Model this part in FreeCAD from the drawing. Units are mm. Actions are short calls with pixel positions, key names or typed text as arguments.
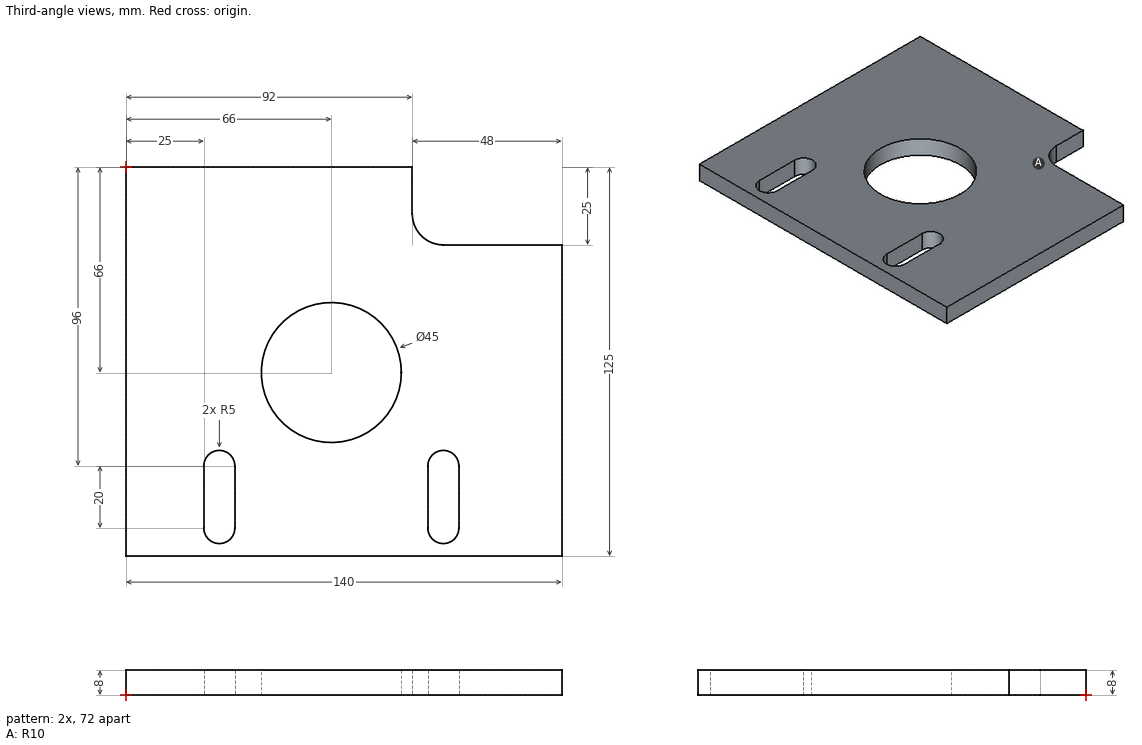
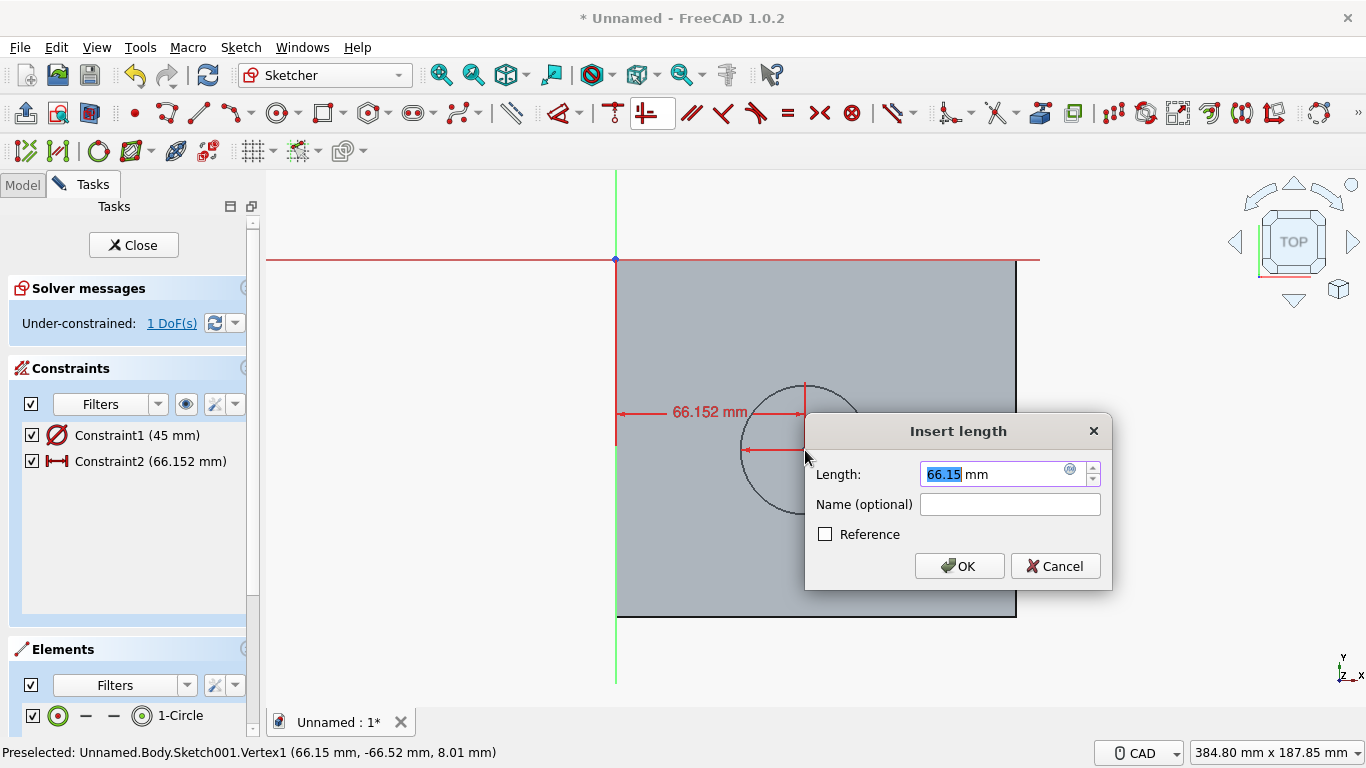
text(66)
key(Return)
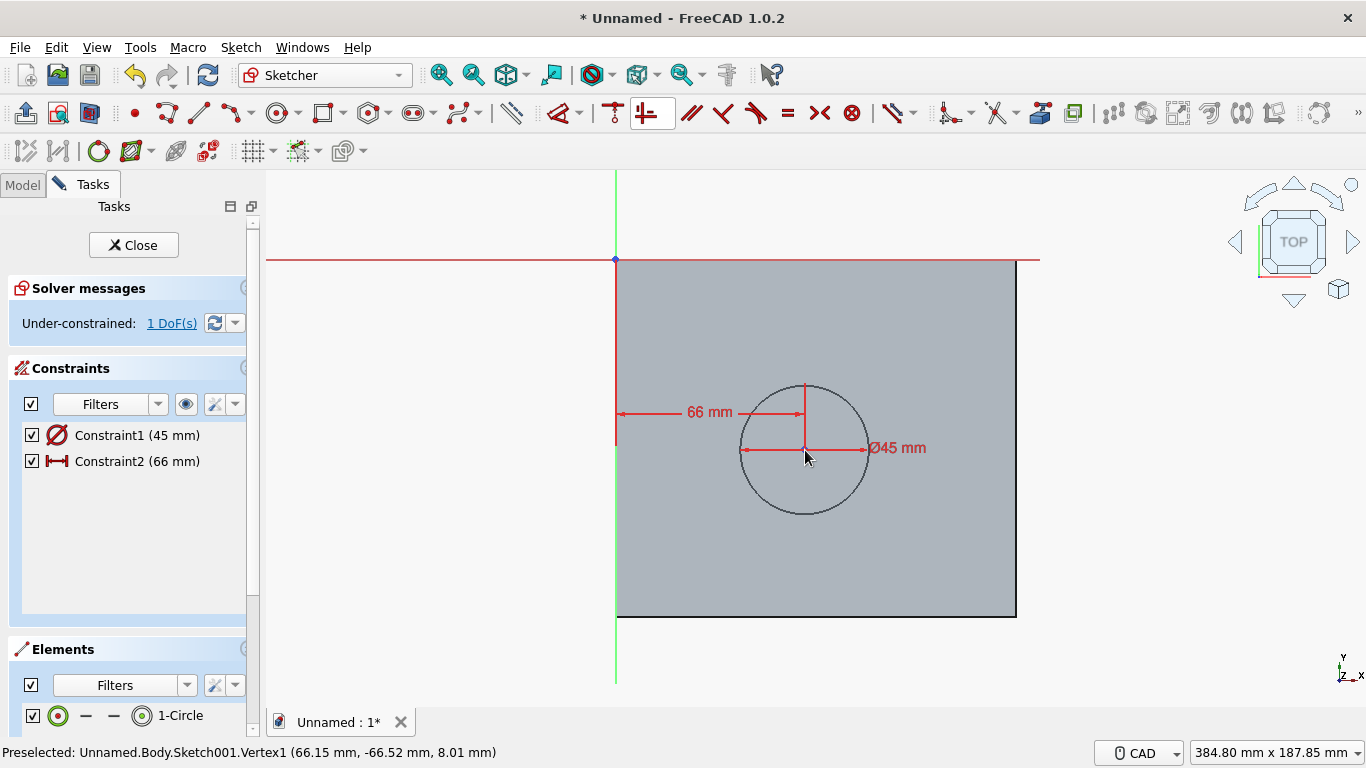
click(805, 450)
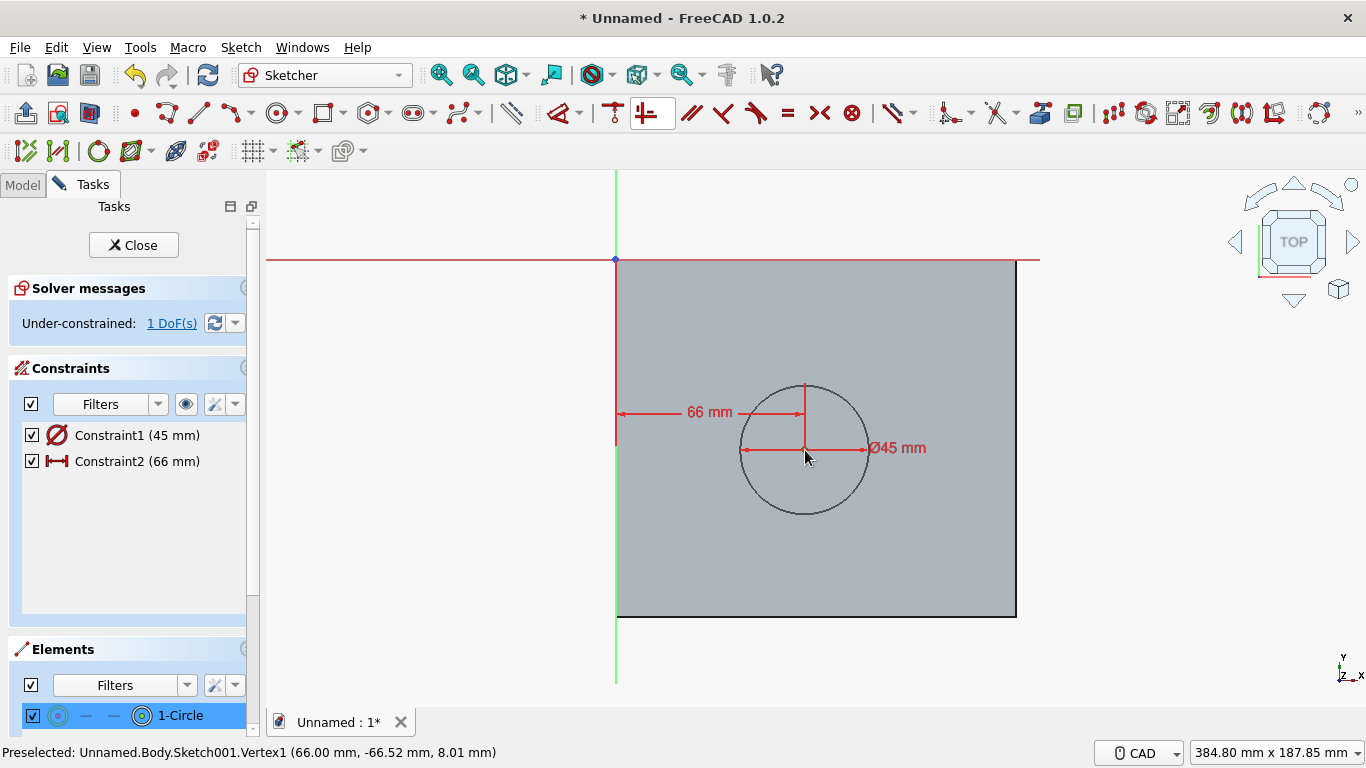
key(i)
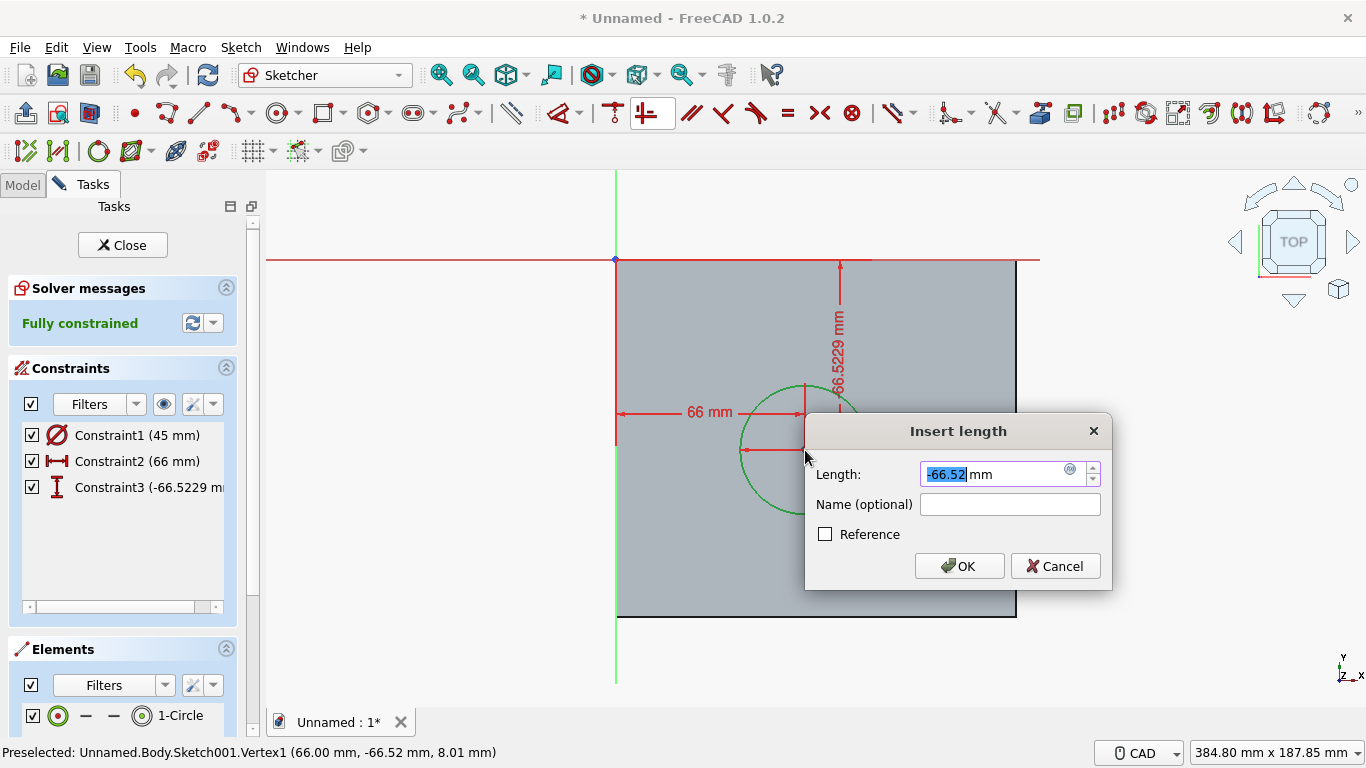
text(-66)
key(Return)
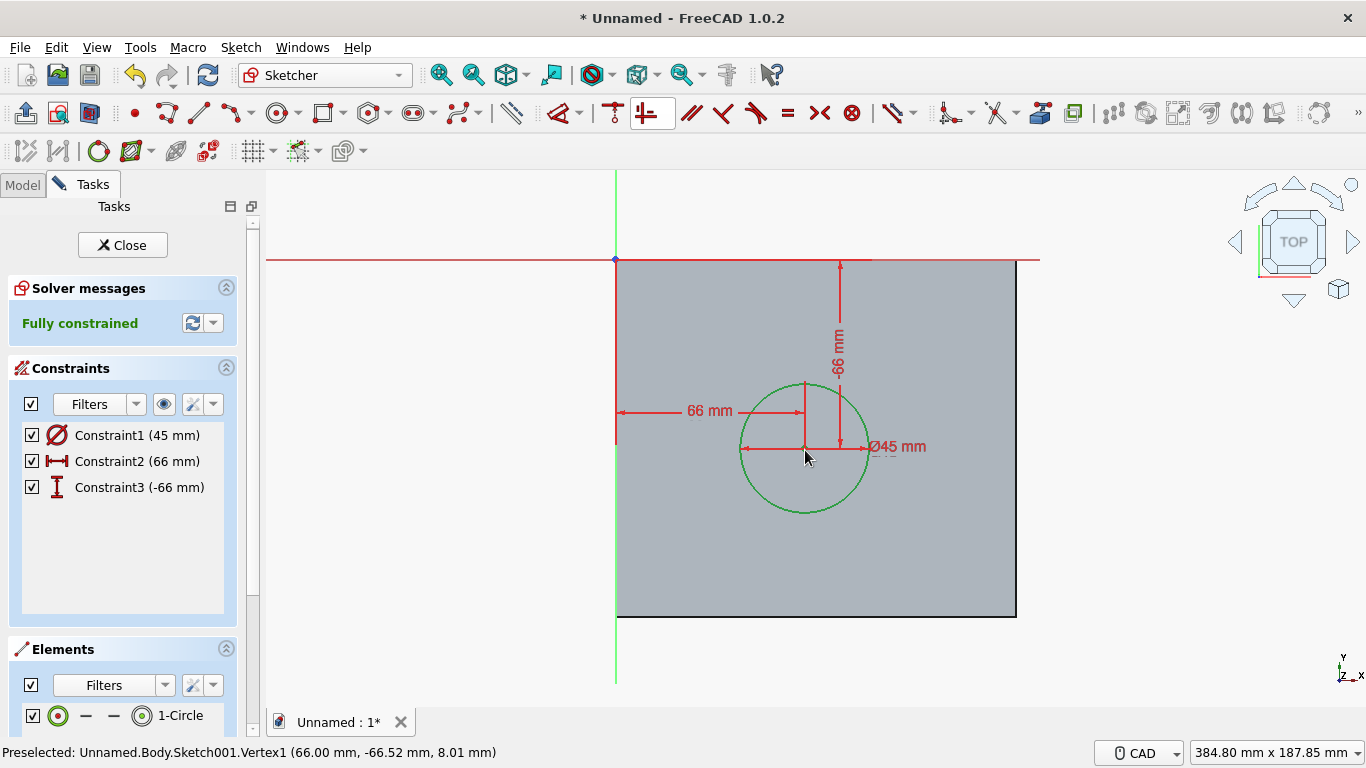
click(123, 245)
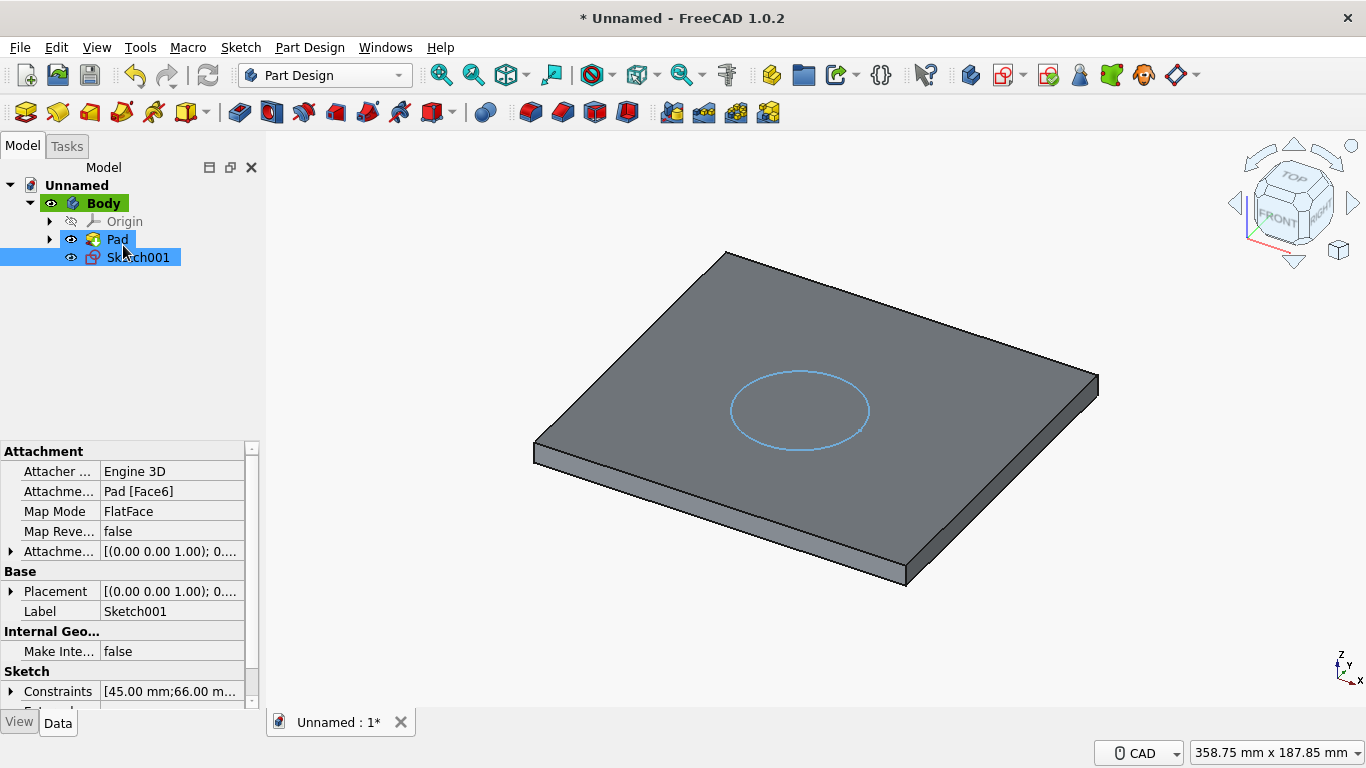
click(240, 112)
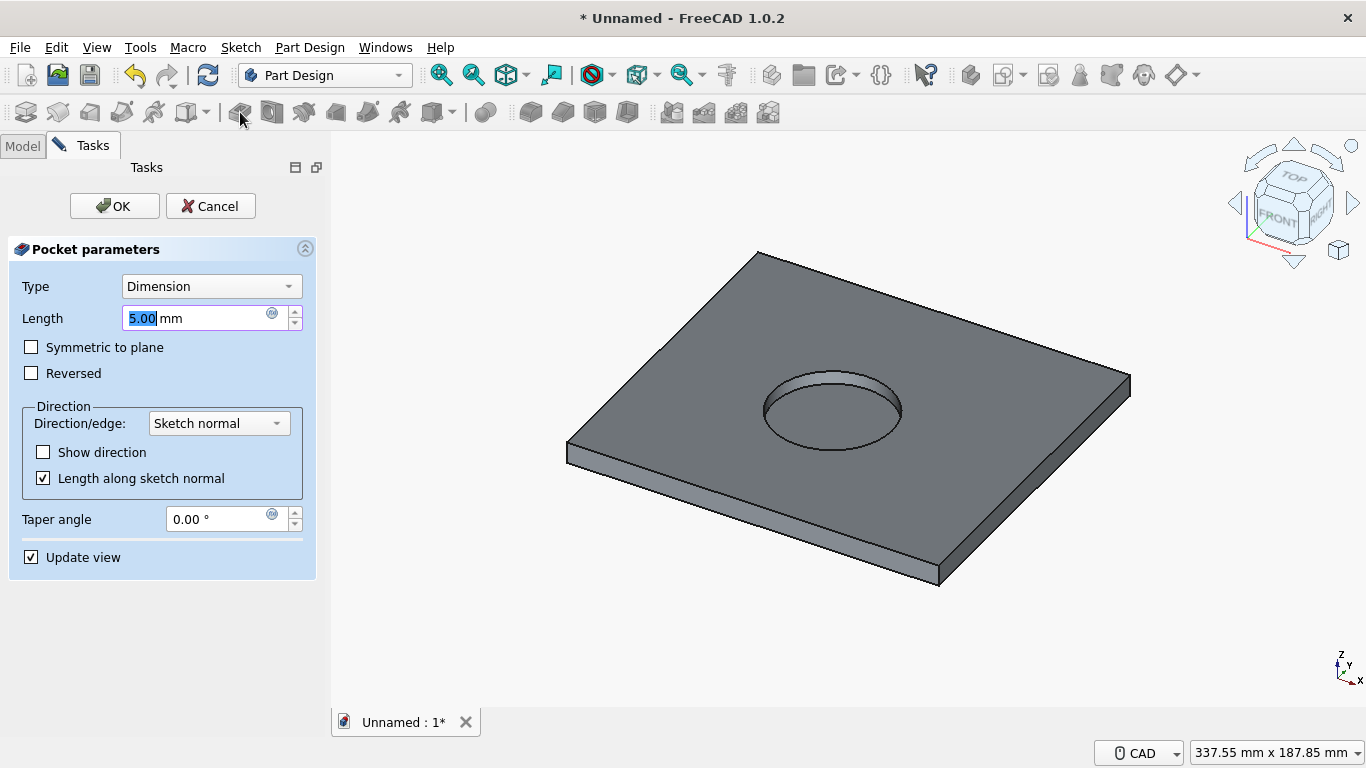
text(8)
key(Tab)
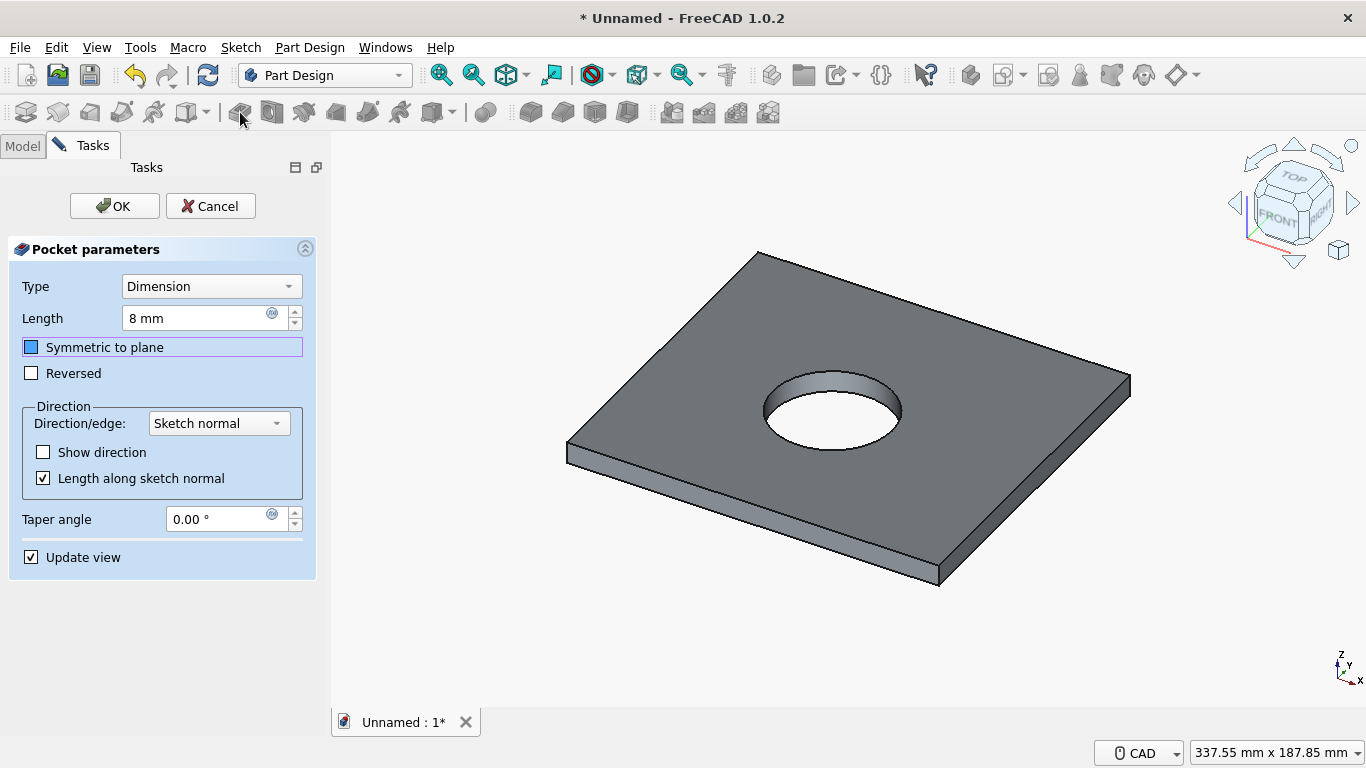
click(115, 206)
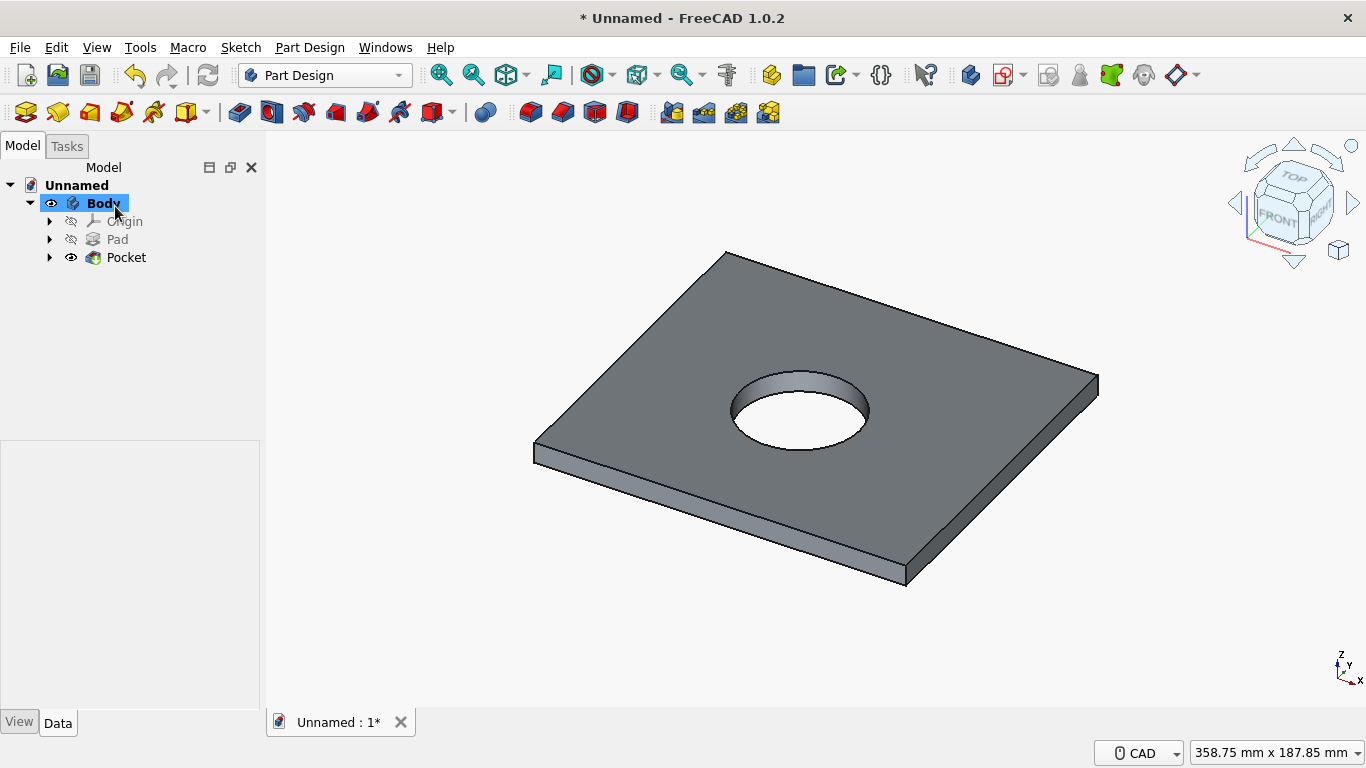
click(977, 389)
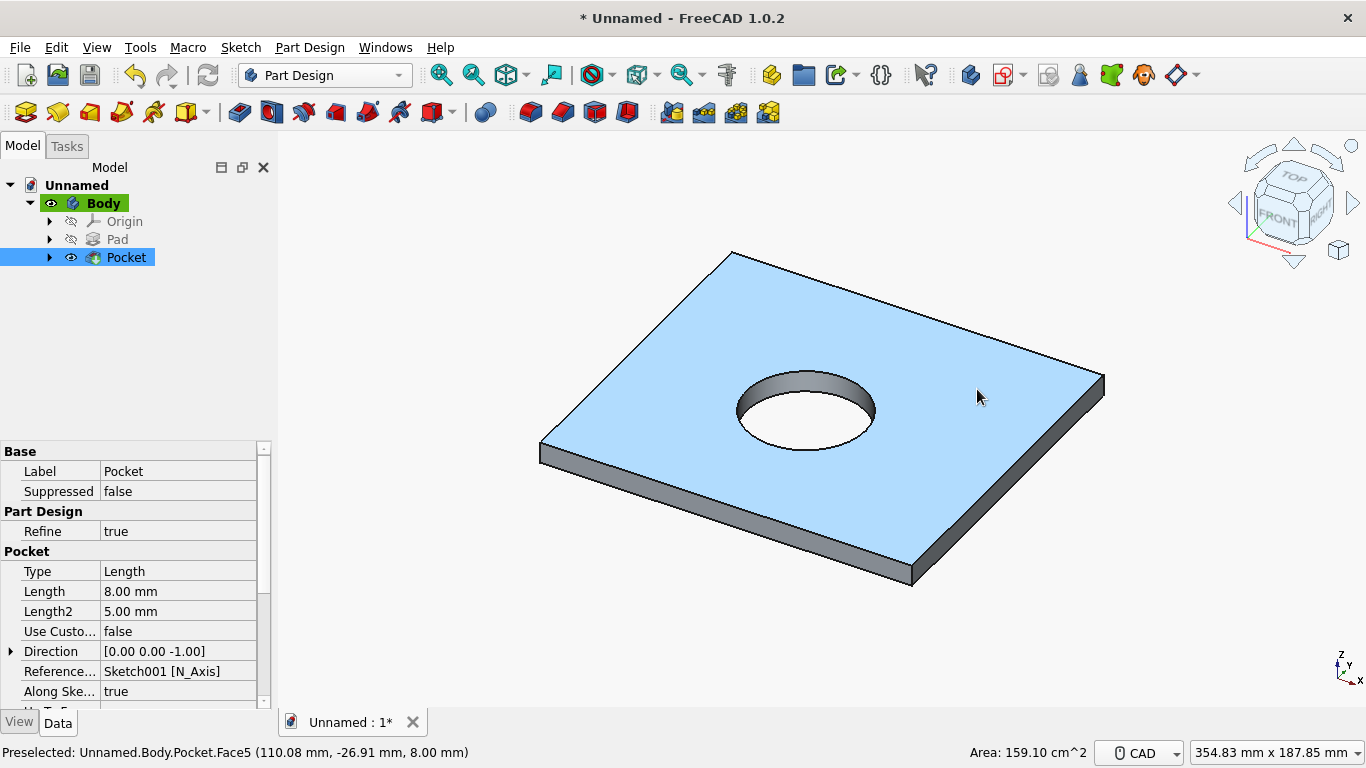
click(1004, 76)